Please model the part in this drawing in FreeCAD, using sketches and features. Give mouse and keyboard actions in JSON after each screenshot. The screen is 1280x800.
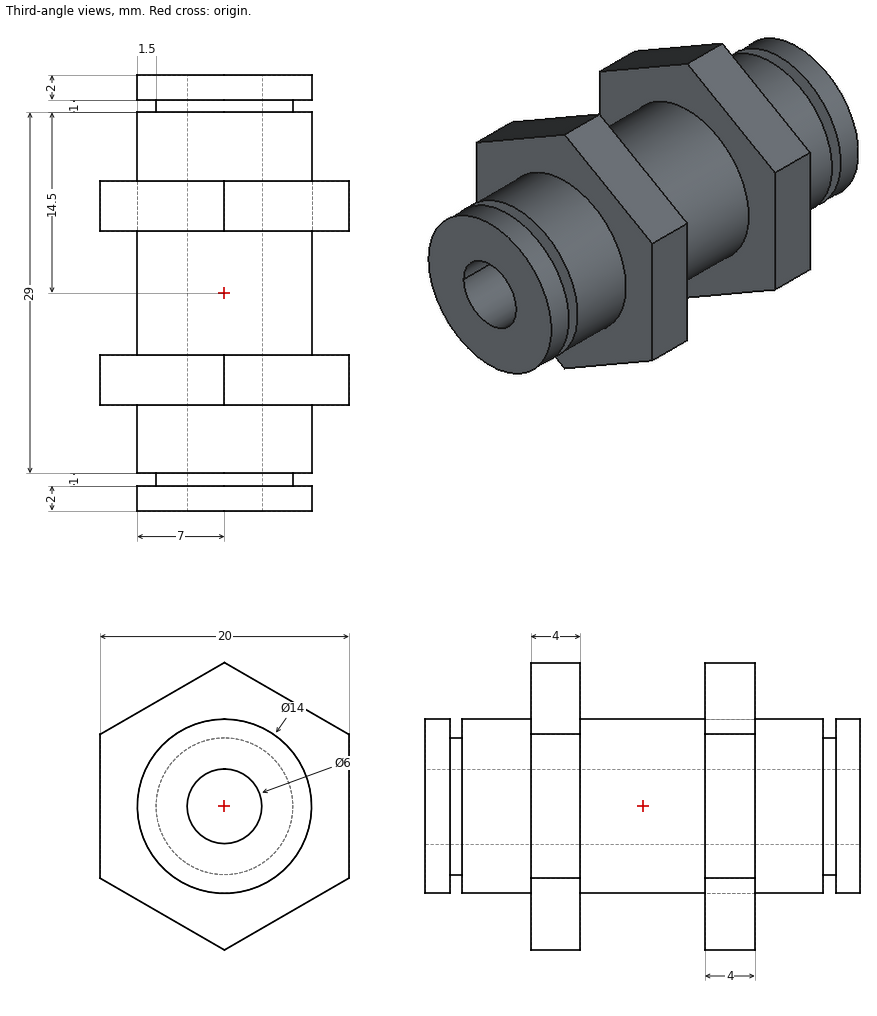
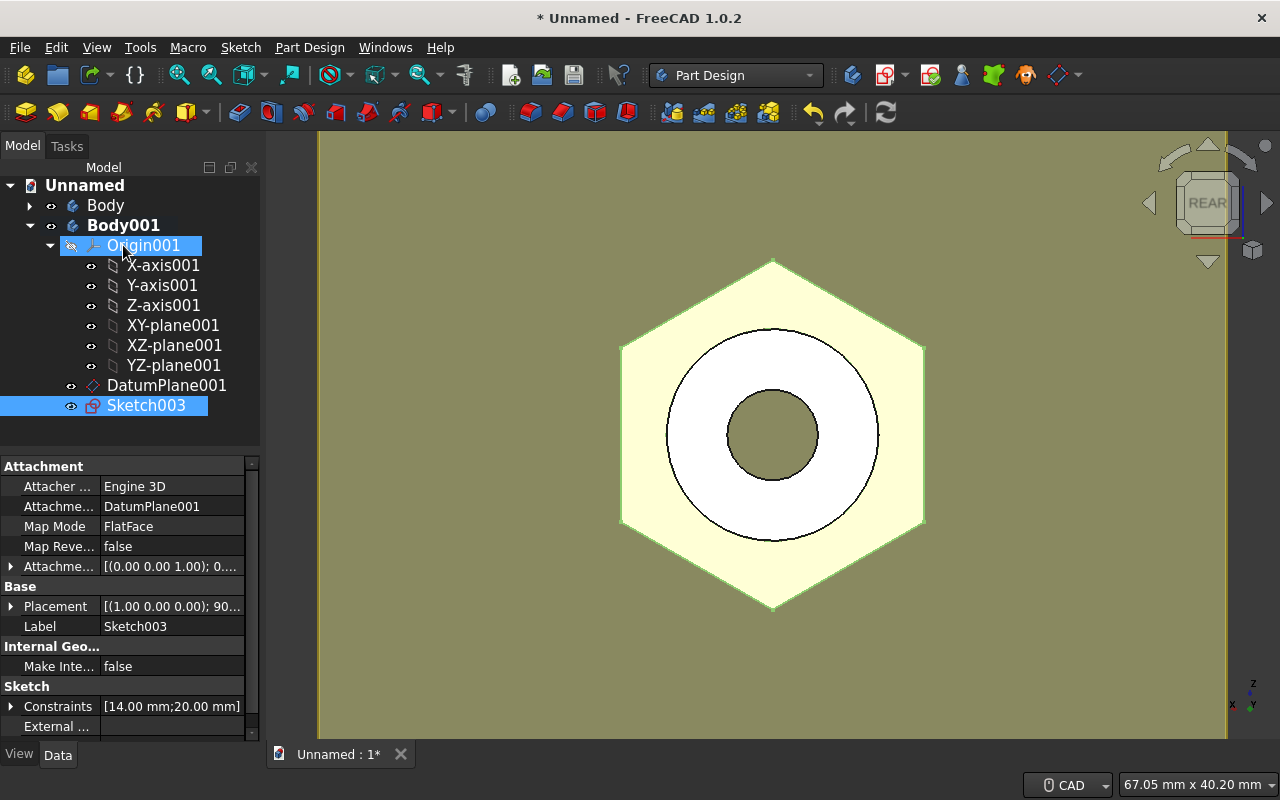
{"action": "left_click", "coordinate": [26, 112]}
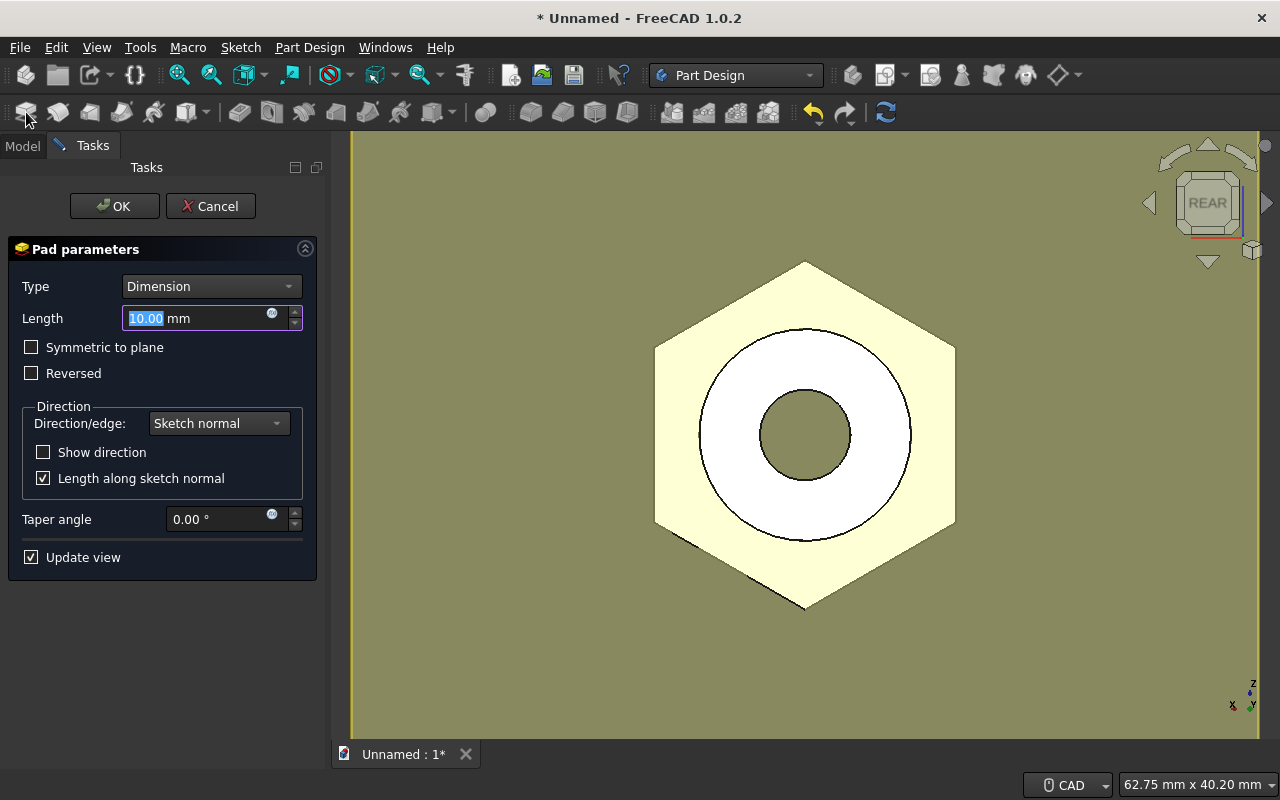
{"action": "type", "text": "4"}
{"action": "key", "text": "Tab"}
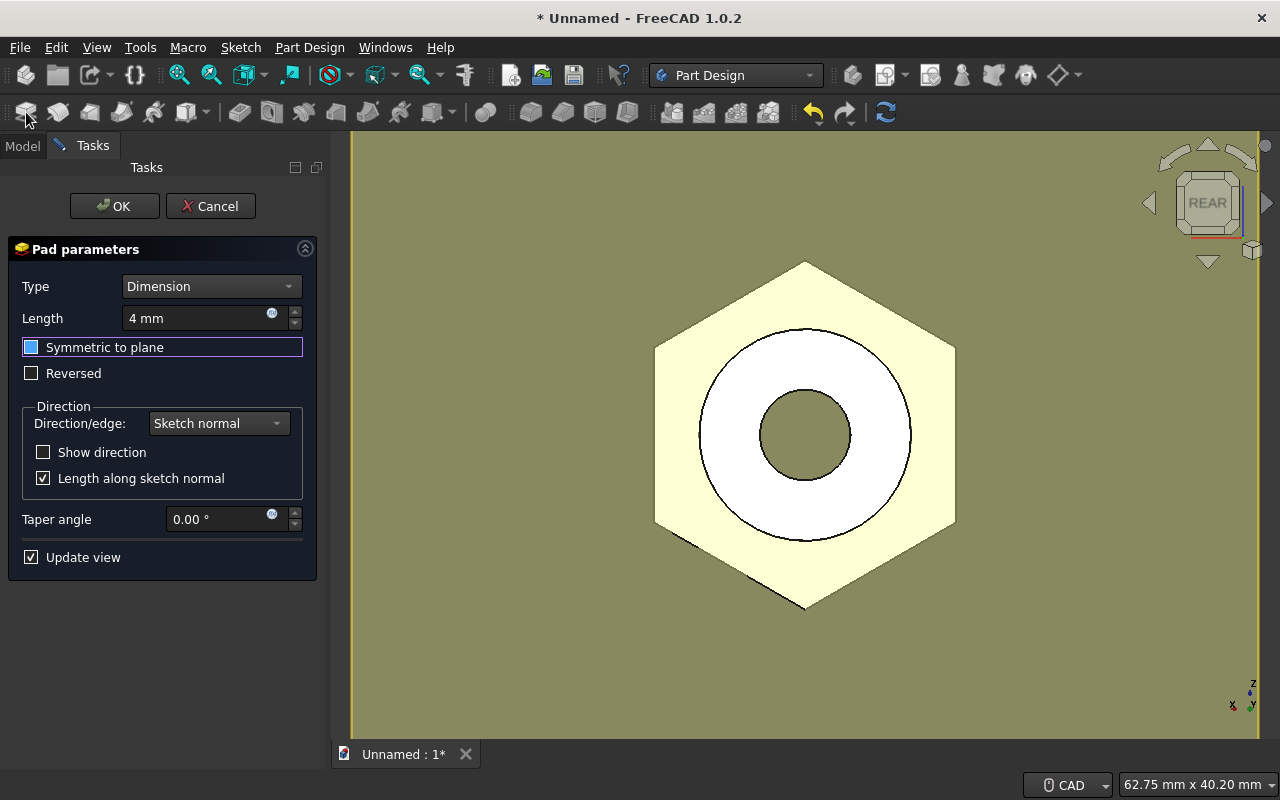
{"action": "left_click", "coordinate": [30, 373]}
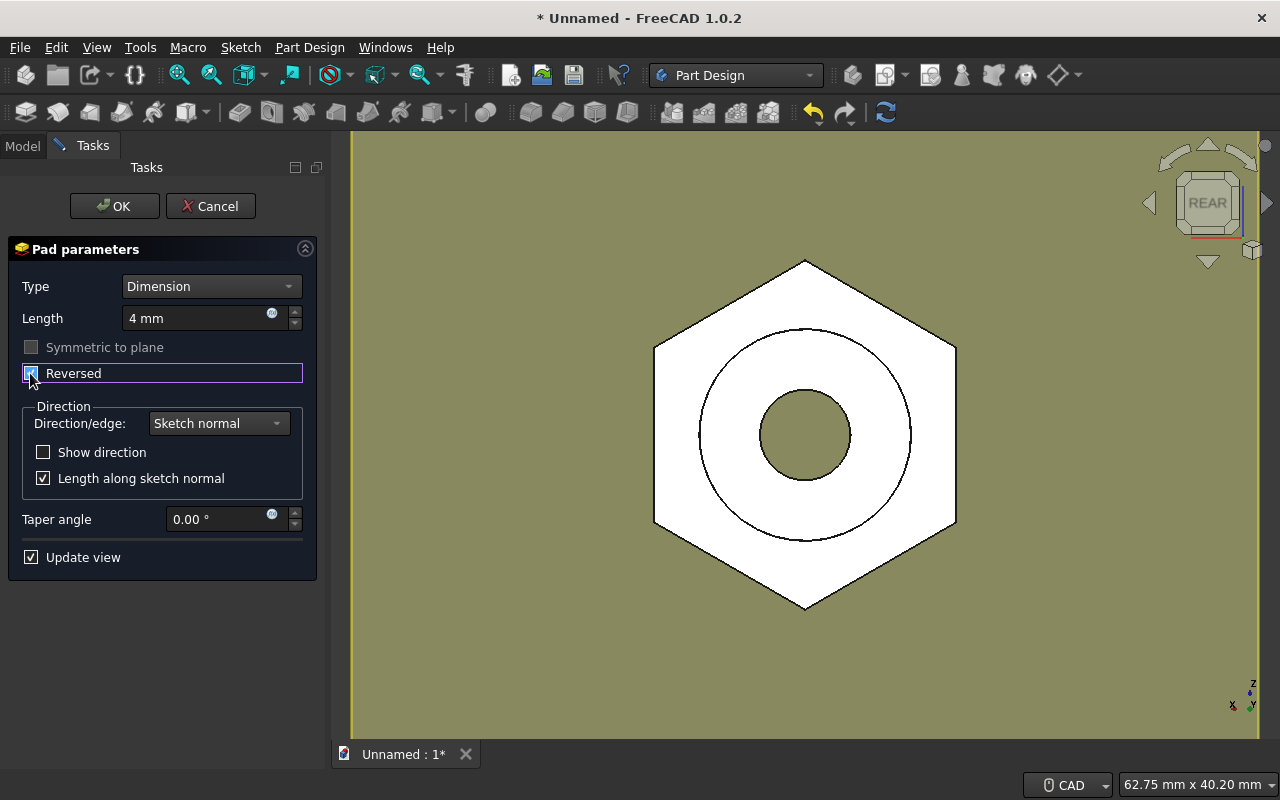
{"action": "left_click", "coordinate": [115, 206]}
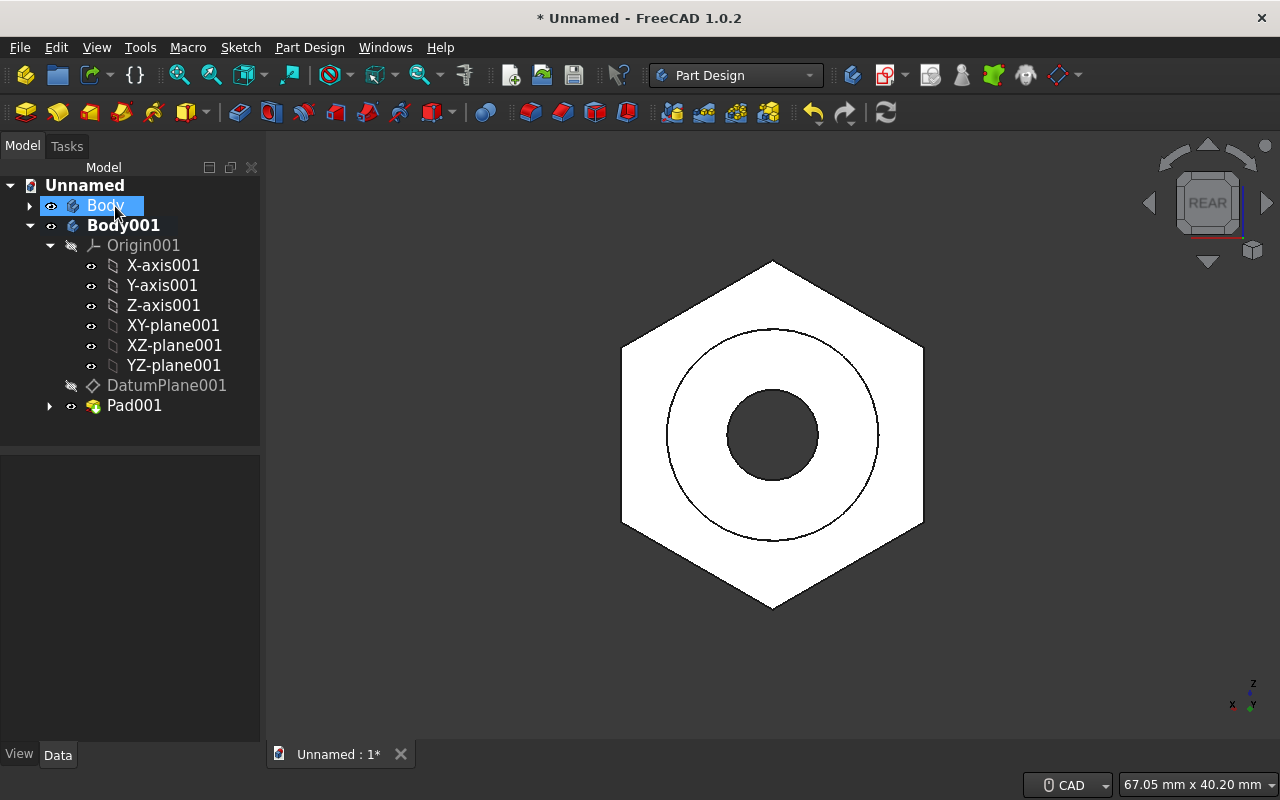
{"action": "key", "text": "0"}